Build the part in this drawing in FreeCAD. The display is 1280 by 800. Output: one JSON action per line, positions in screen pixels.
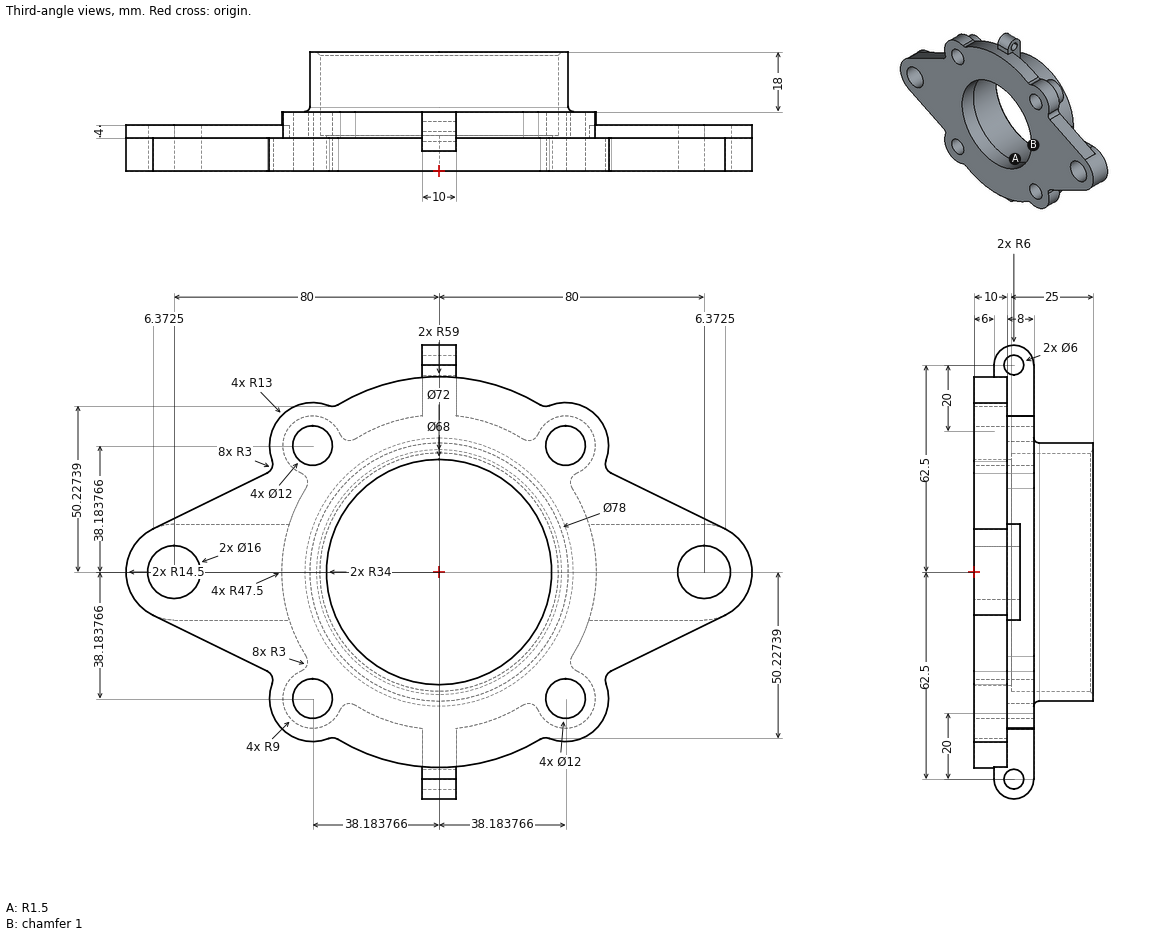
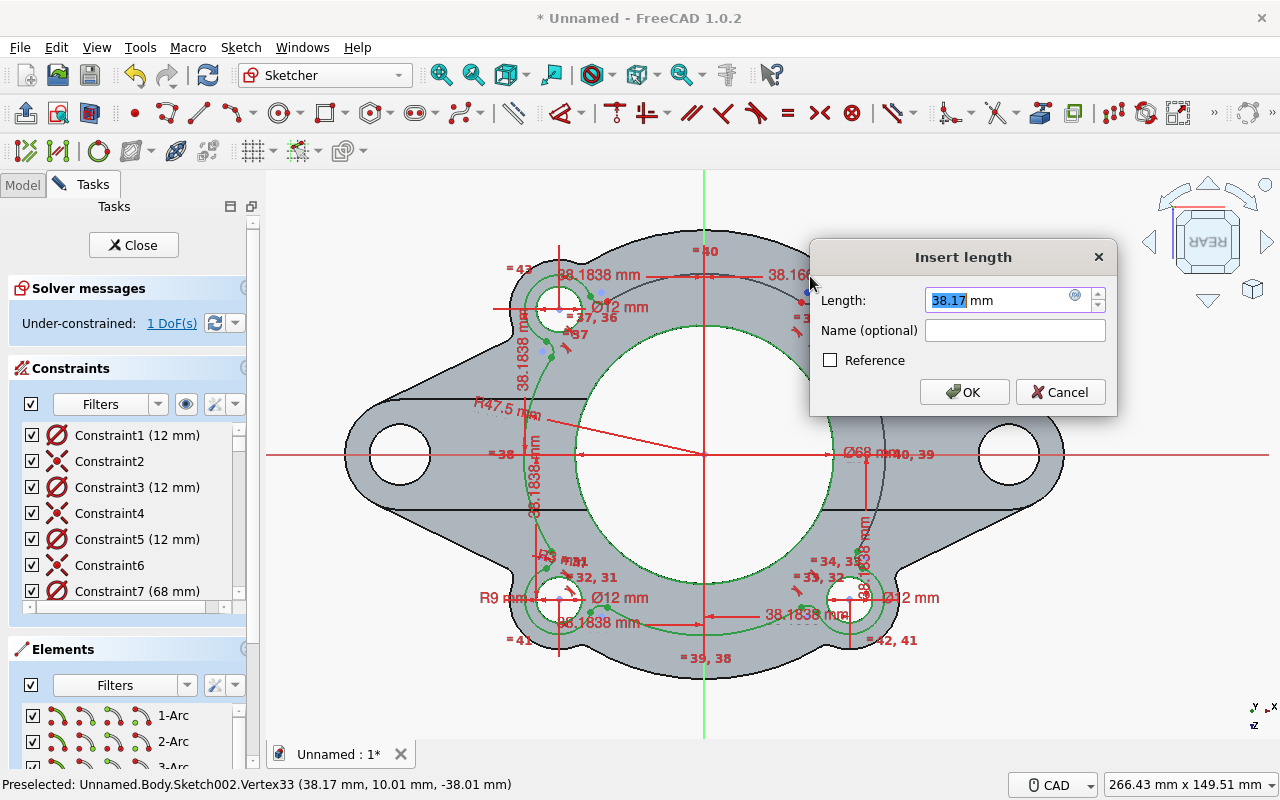
{"action": "type", "text": "38.183766"}
{"action": "key", "text": "Return"}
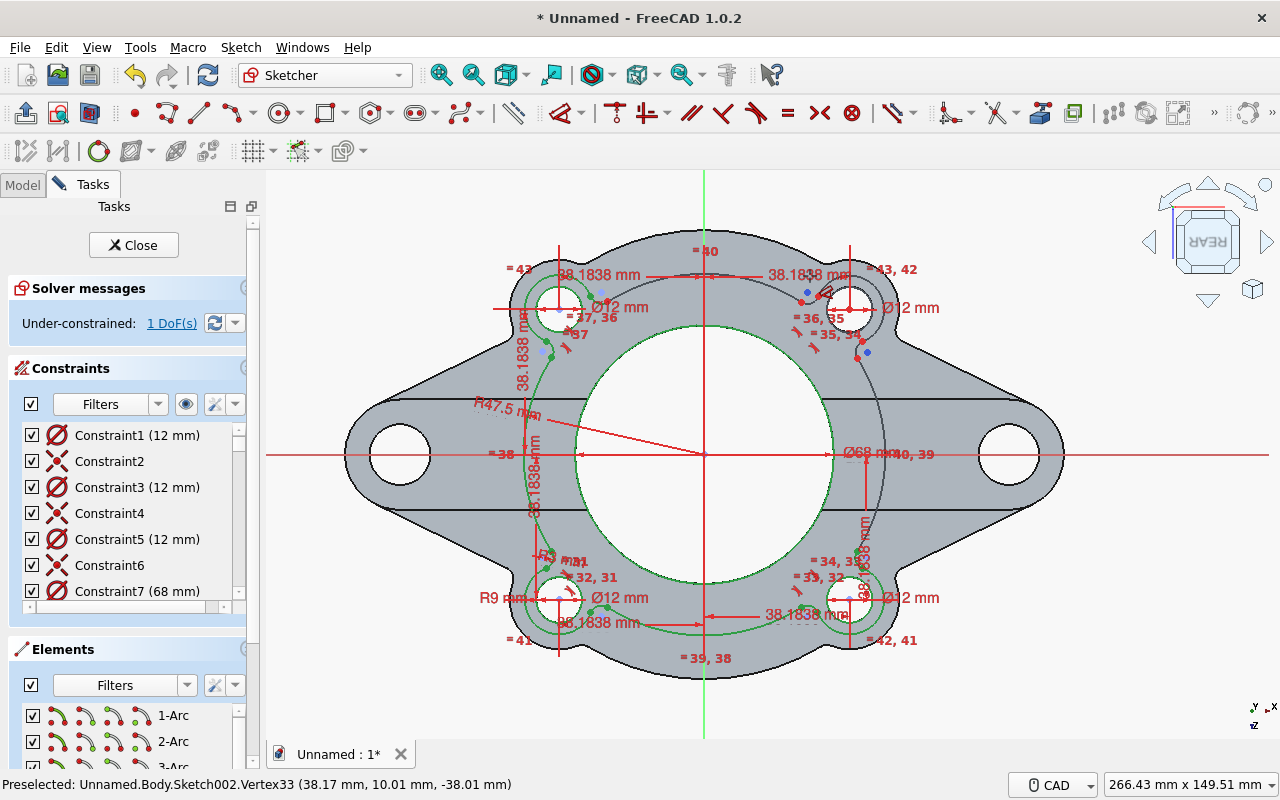
{"action": "left_click", "coordinate": [850, 310]}
{"action": "left_click", "coordinate": [884, 349]}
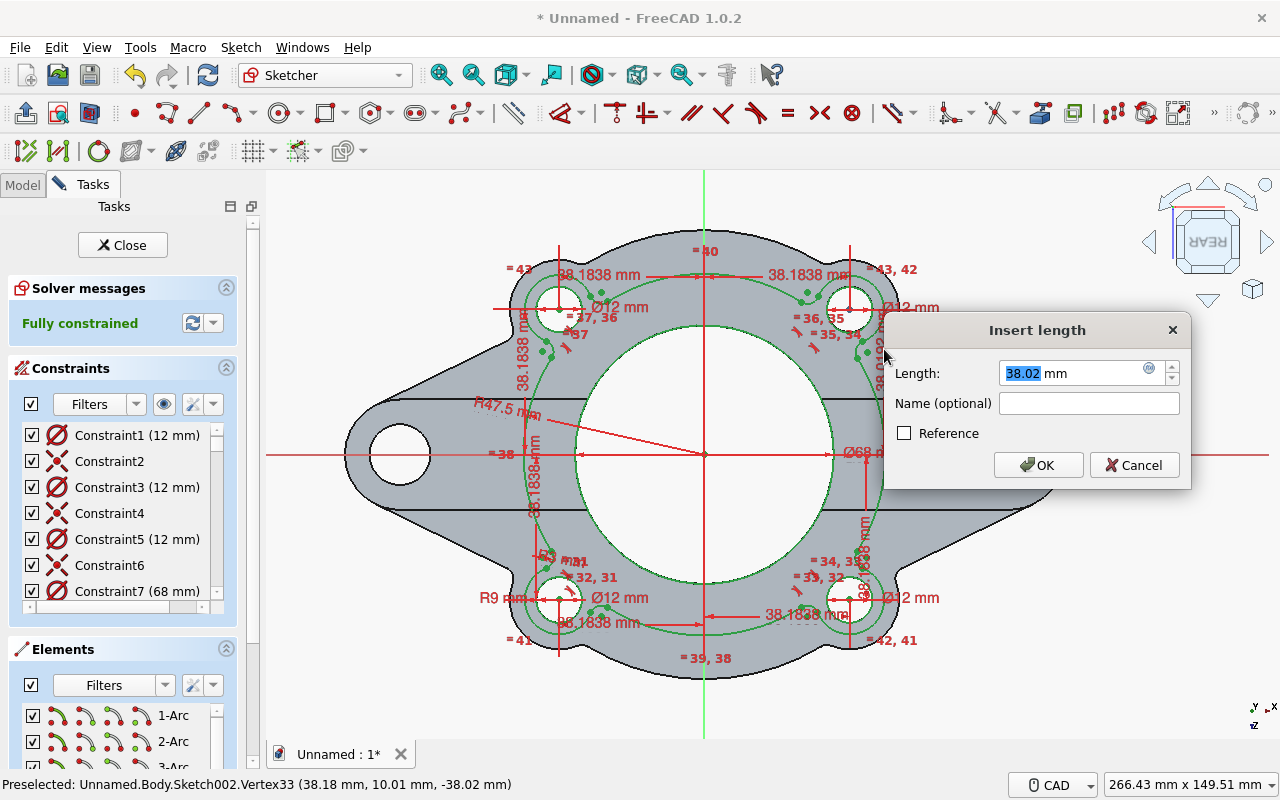
{"action": "type", "text": "38.183766"}
{"action": "key", "text": "Return"}
{"action": "key", "text": "Escape"}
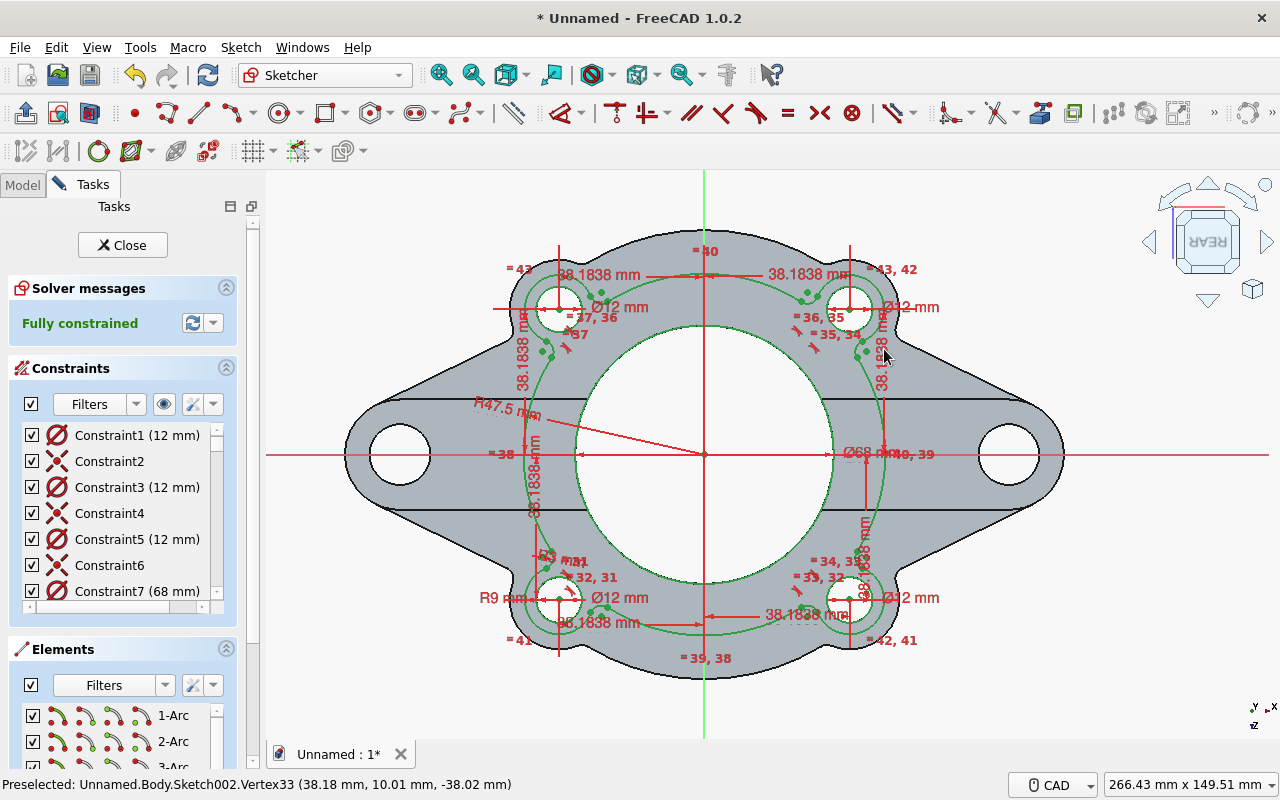
{"action": "left_click", "coordinate": [123, 245]}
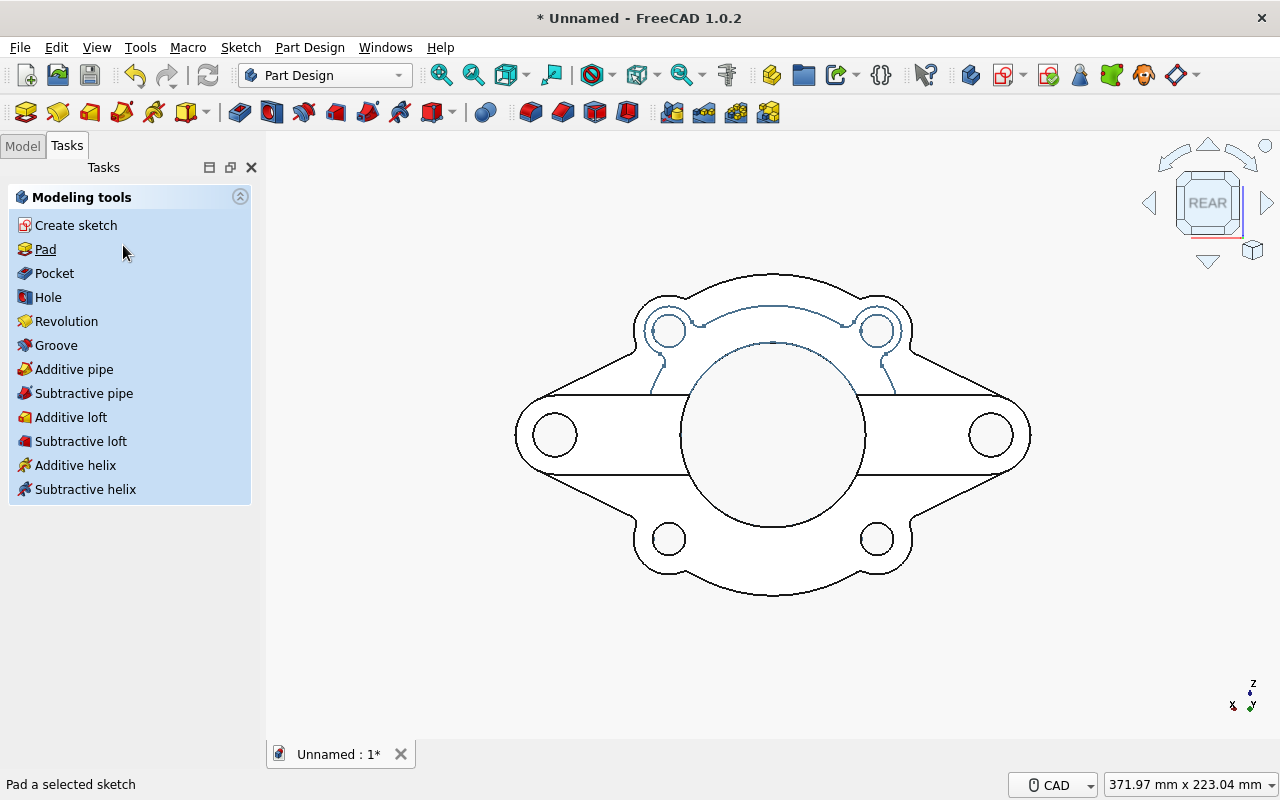
{"action": "left_click", "coordinate": [26, 112]}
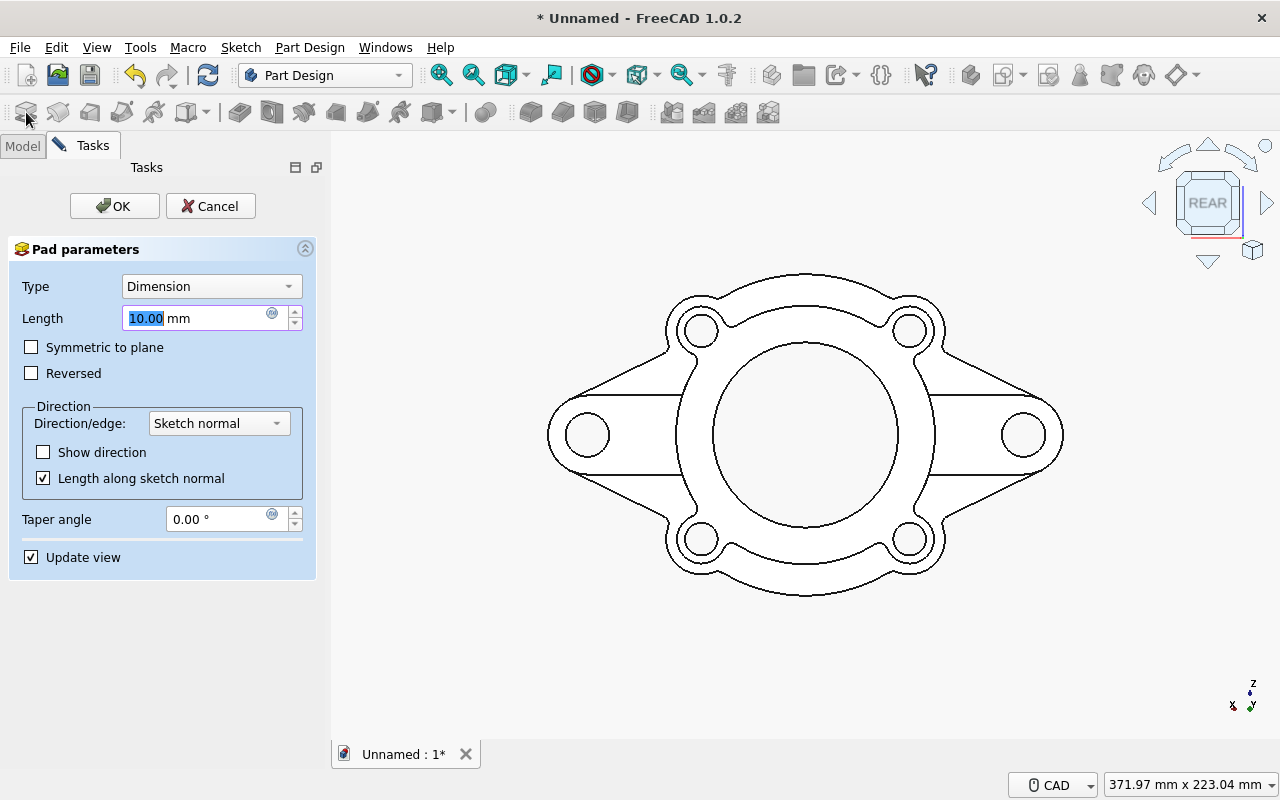
{"action": "type", "text": "8"}
{"action": "key", "text": "Tab"}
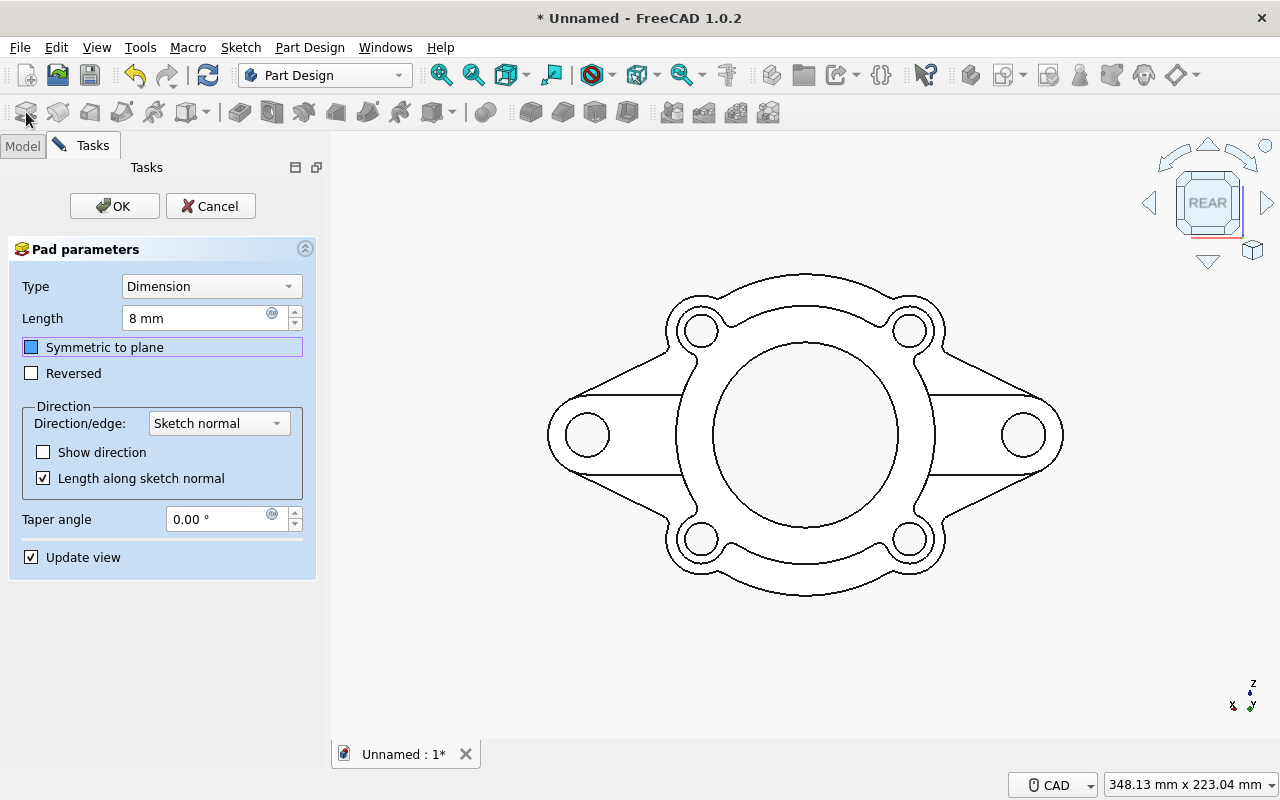
{"action": "left_click", "coordinate": [115, 206]}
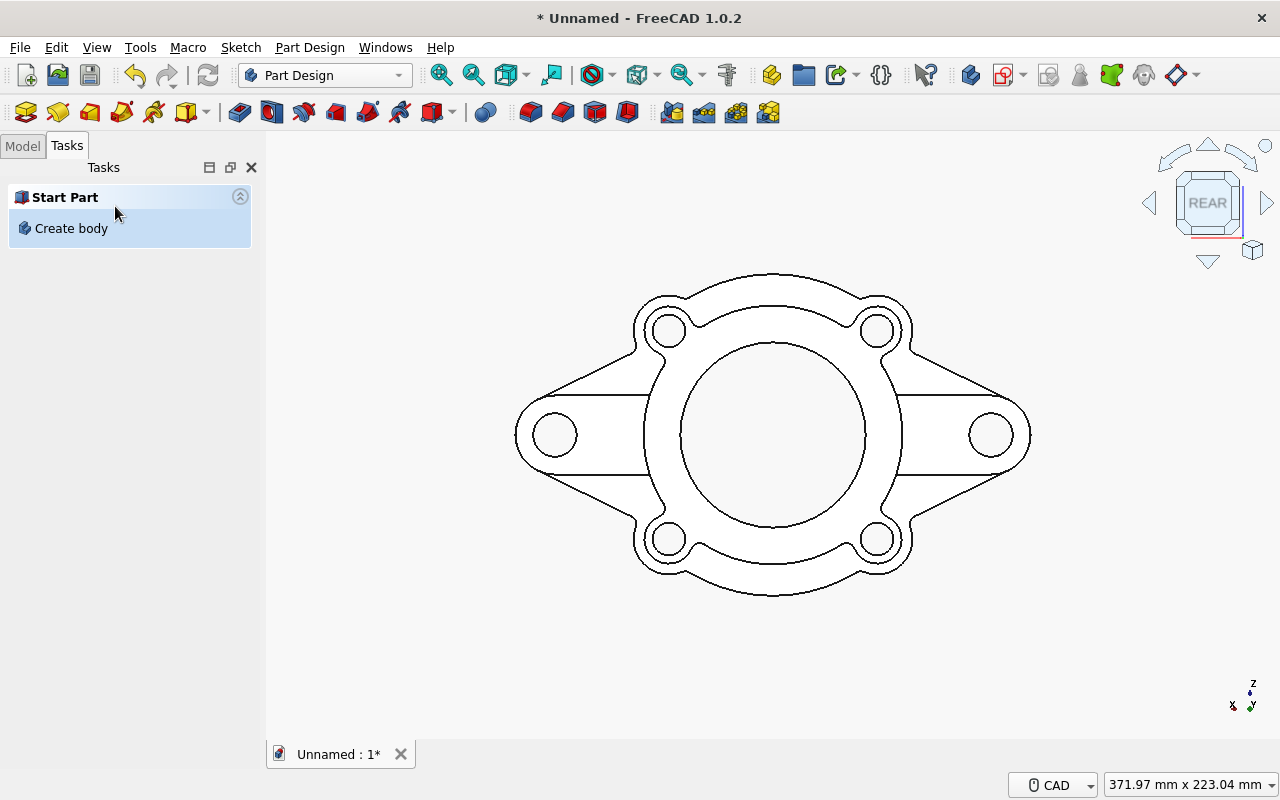
{"action": "left_click", "coordinate": [773, 545]}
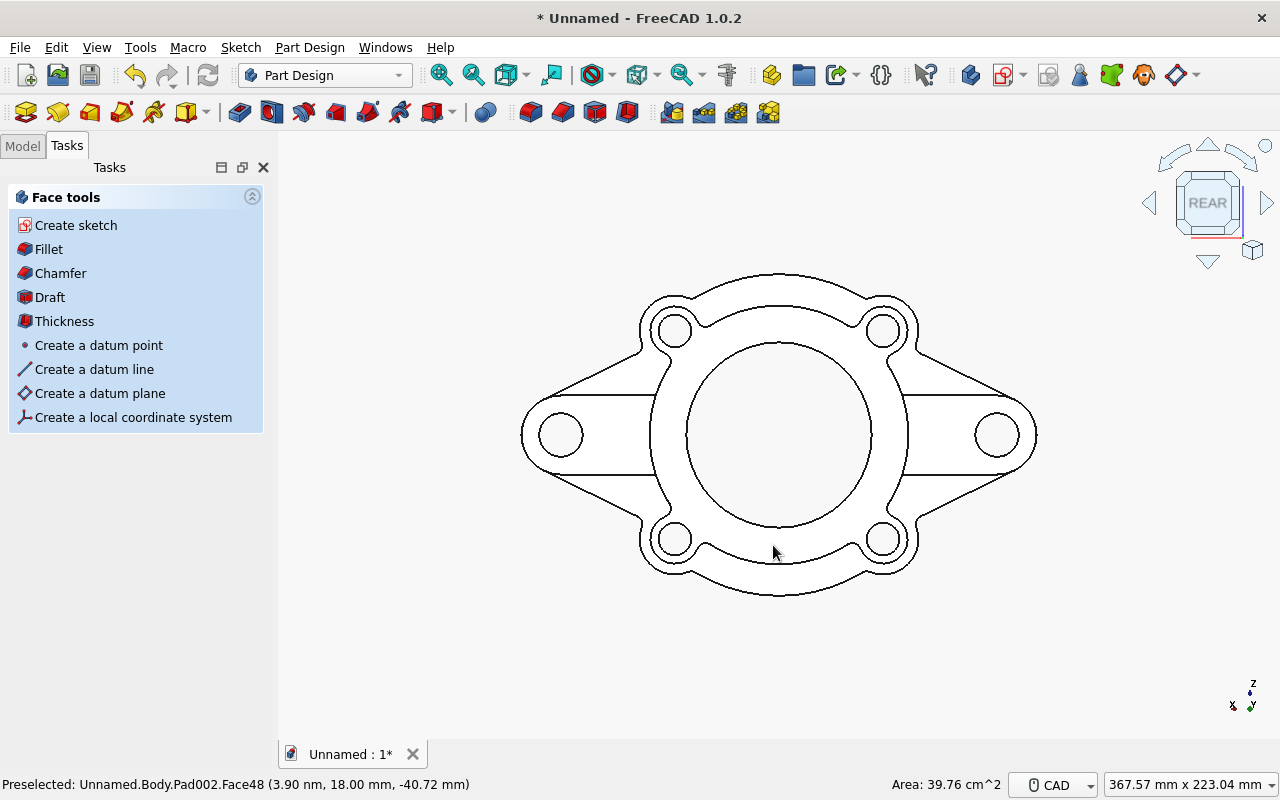
{"action": "left_click", "coordinate": [1004, 76]}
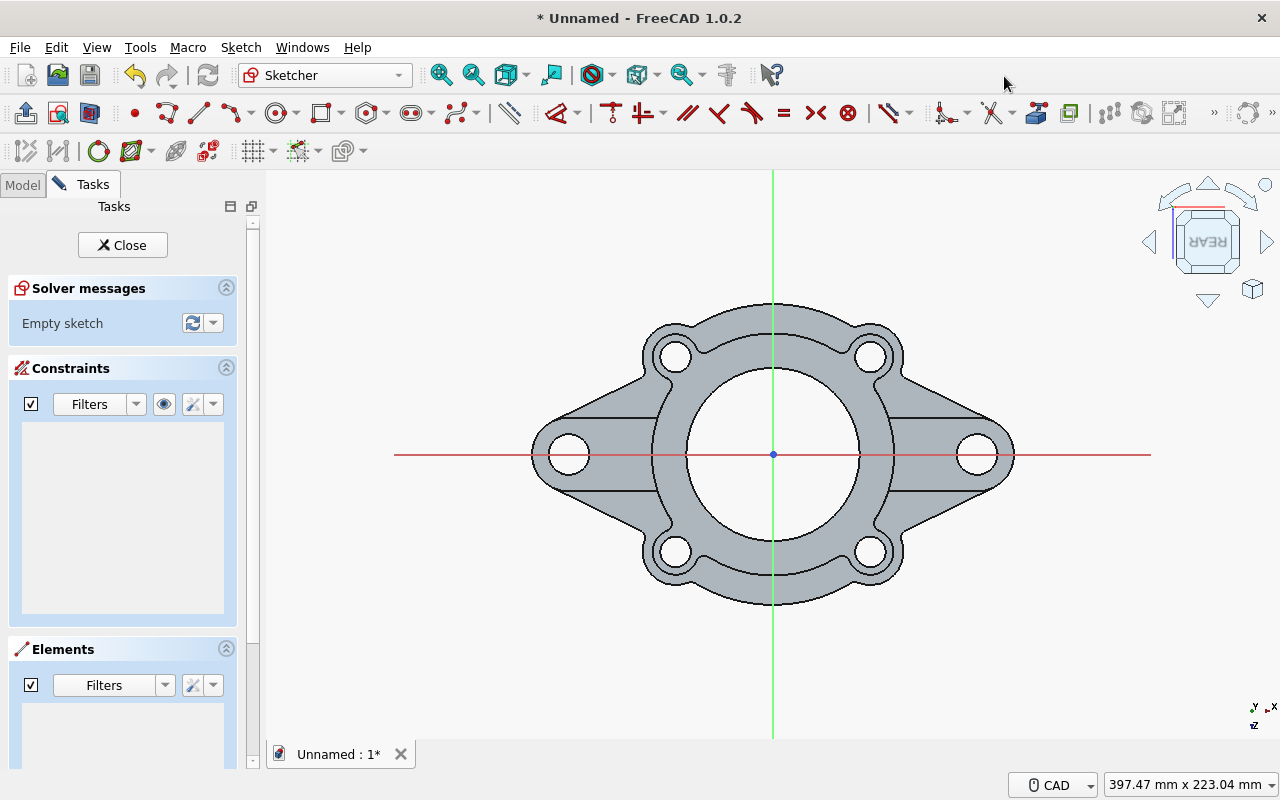
{"action": "scroll", "coordinate": [856, 454], "scroll_direction": "up", "scroll_amount": 3}